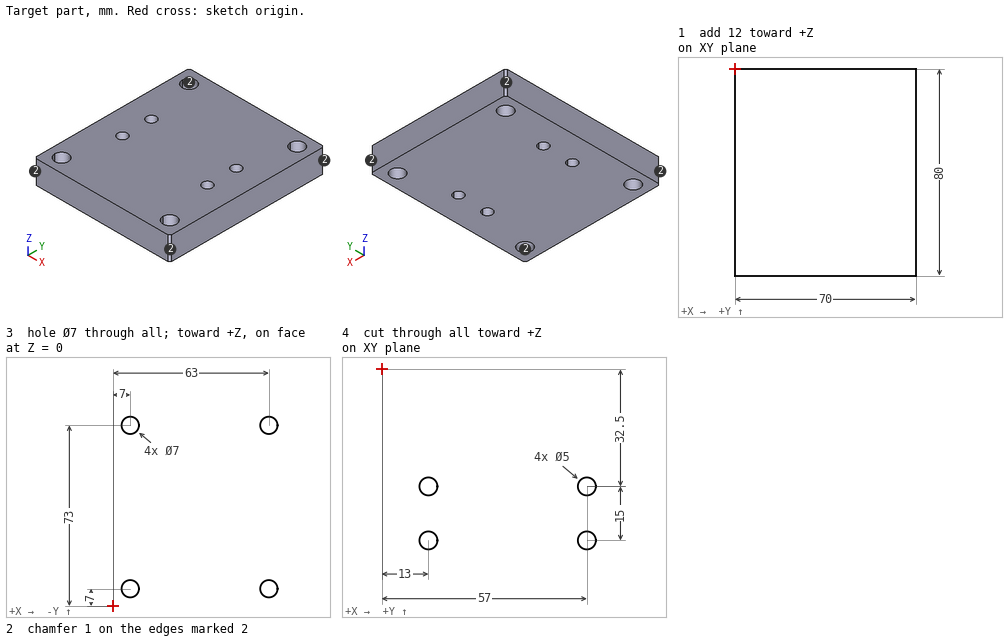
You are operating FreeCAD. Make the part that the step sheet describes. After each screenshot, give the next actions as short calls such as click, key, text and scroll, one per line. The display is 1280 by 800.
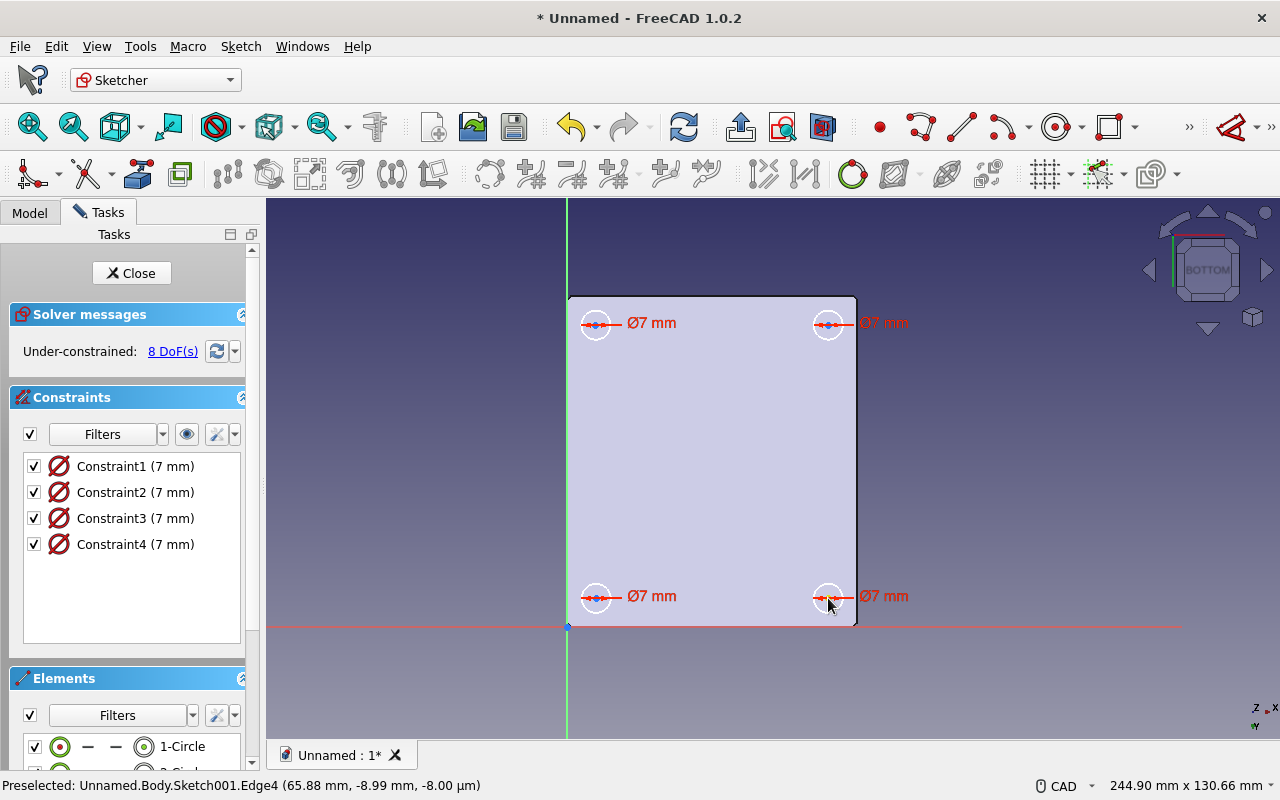
click(596, 325)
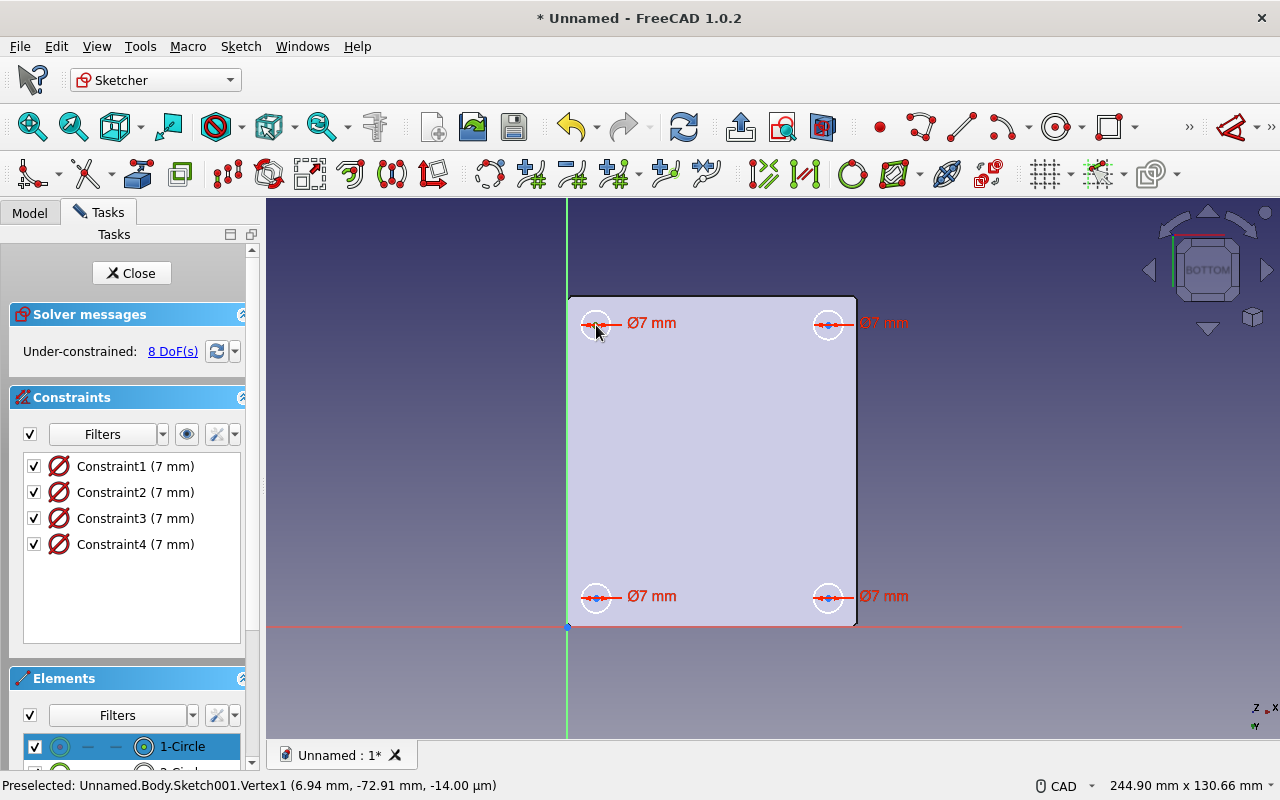
click(596, 598)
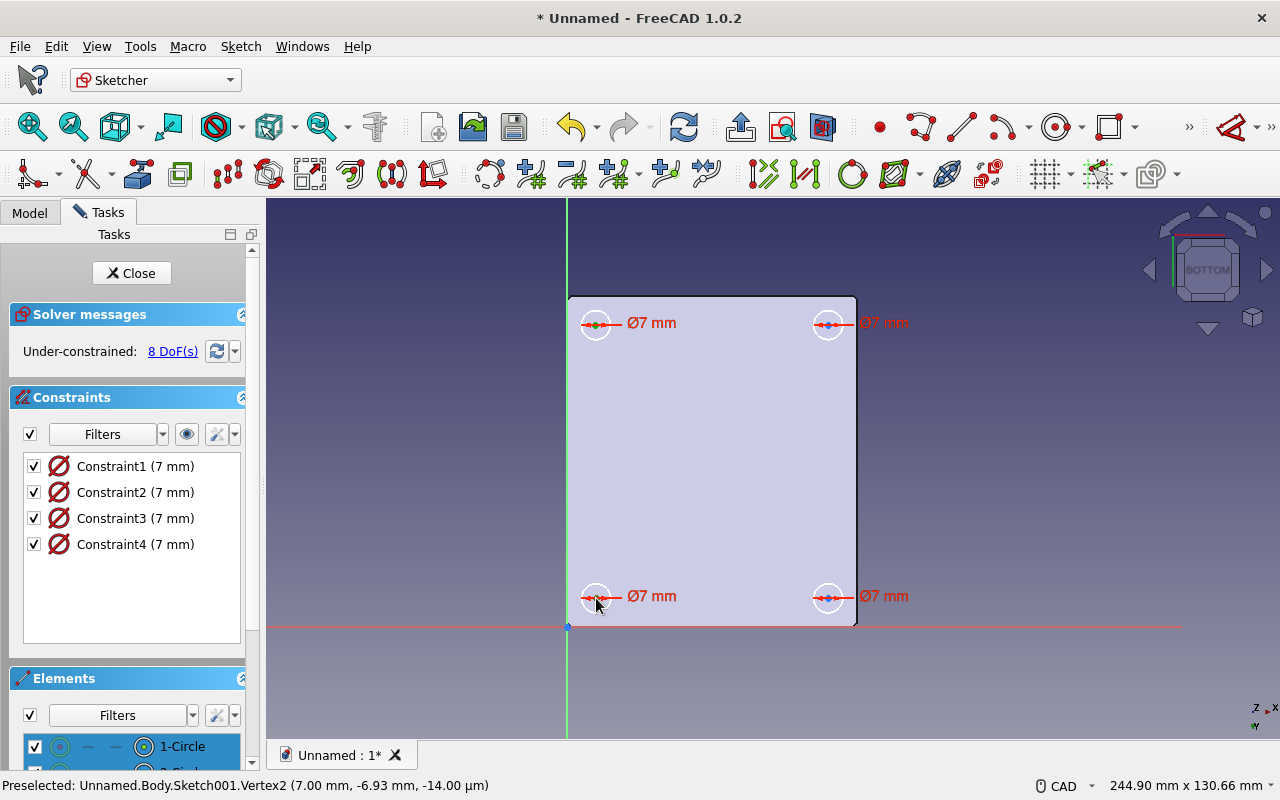
key(v)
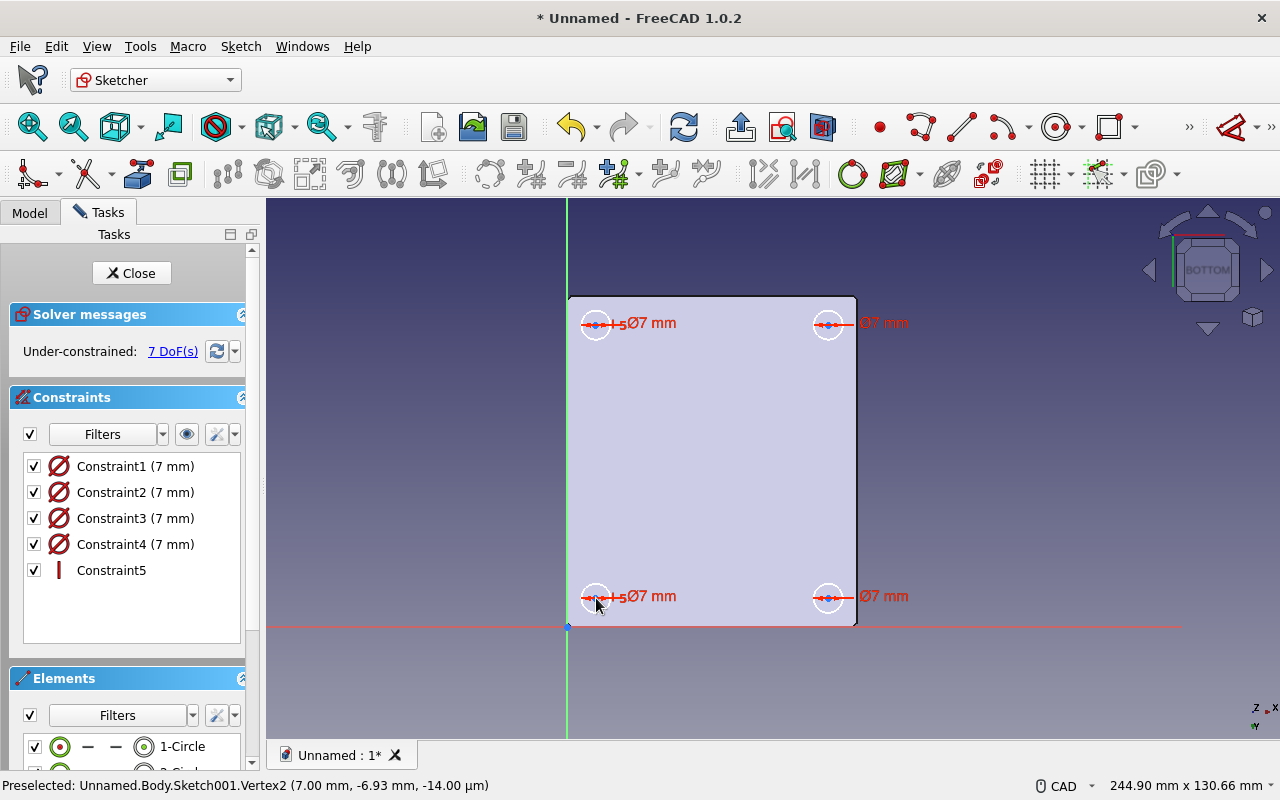
click(596, 325)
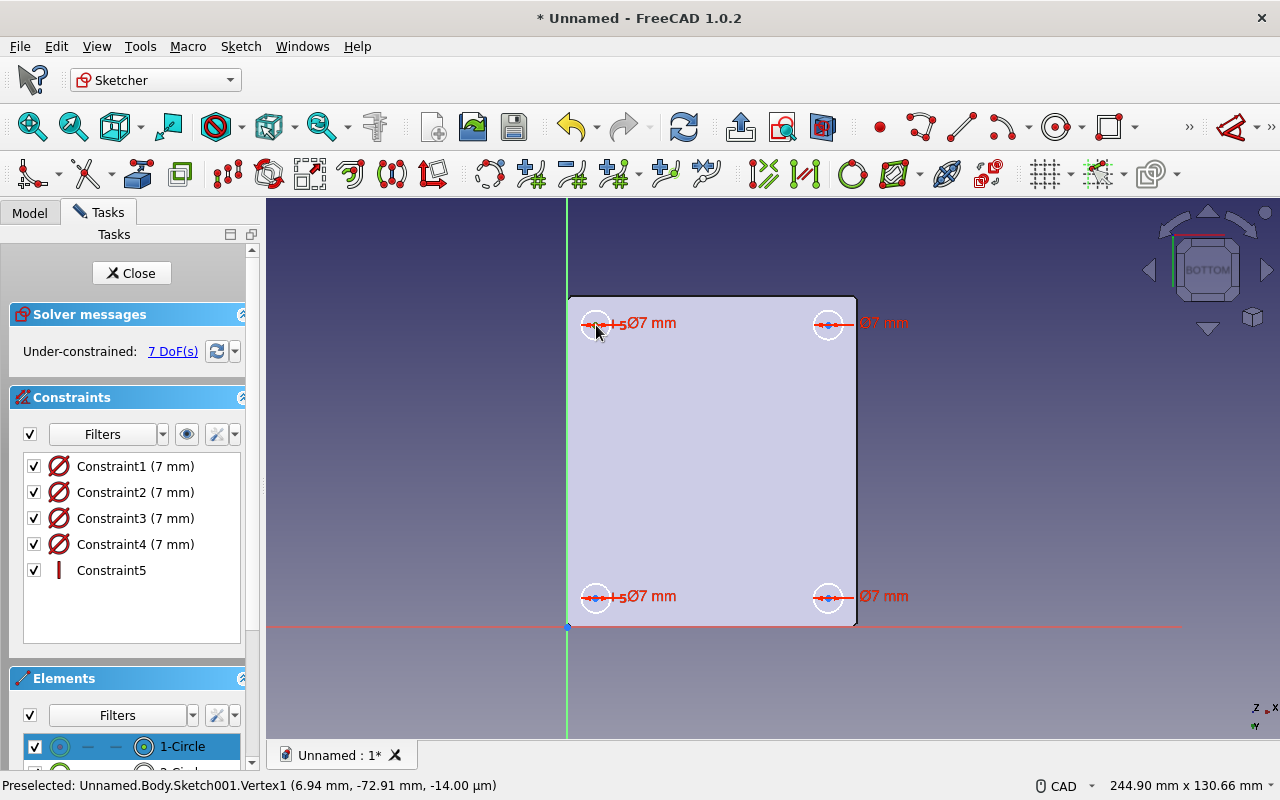
click(828, 325)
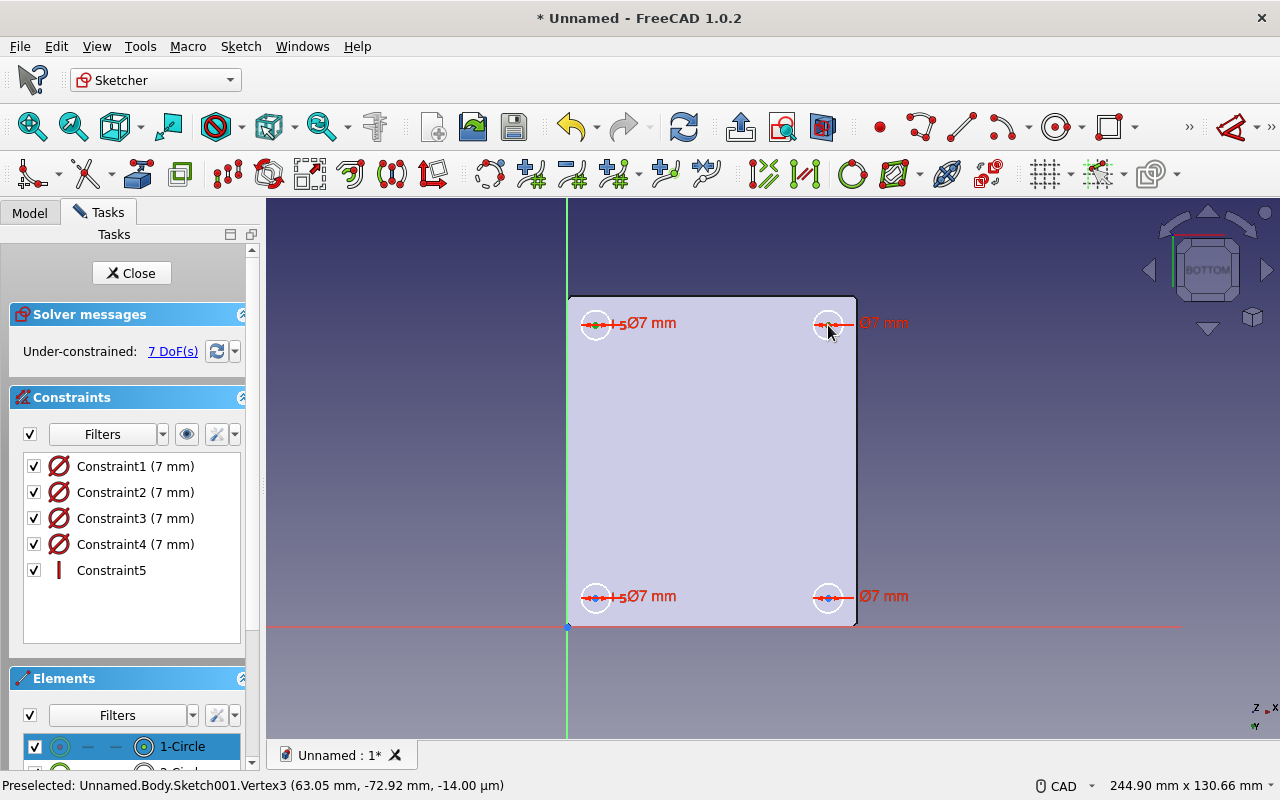
key(h)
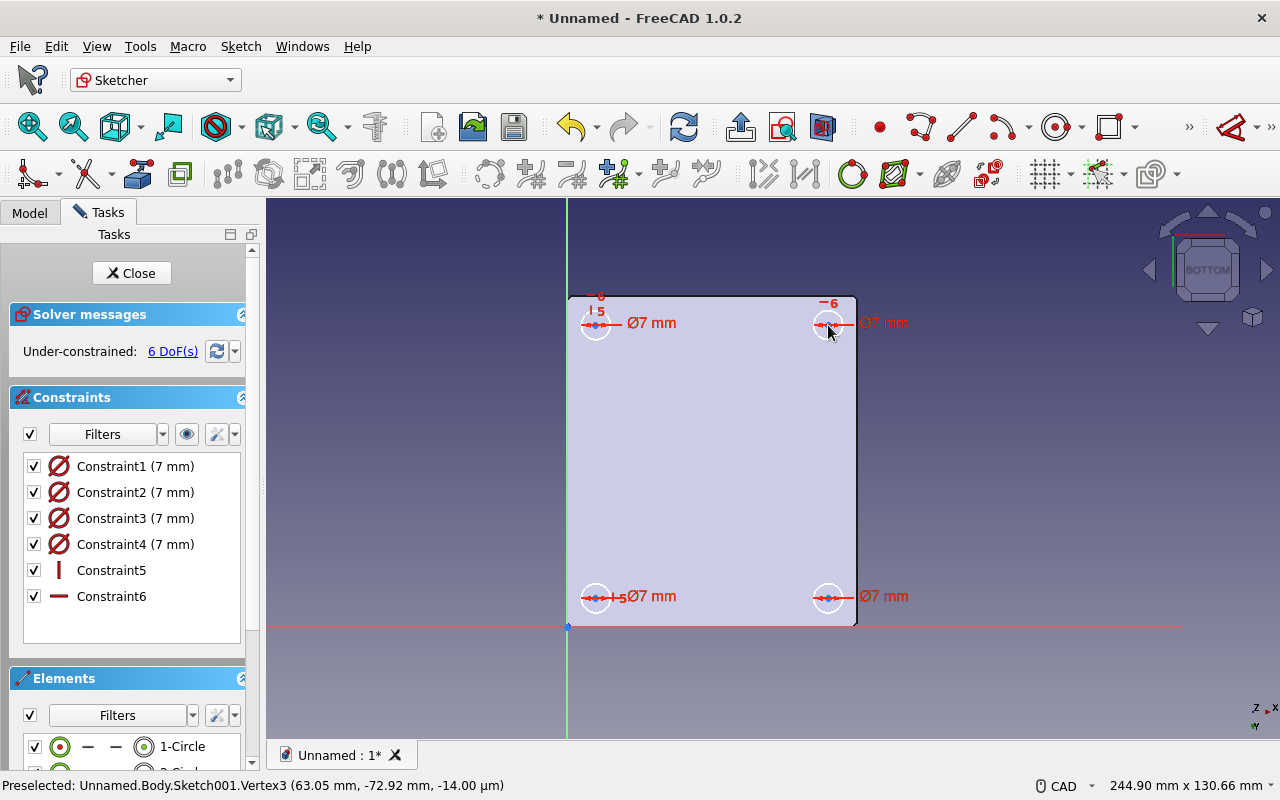
click(828, 325)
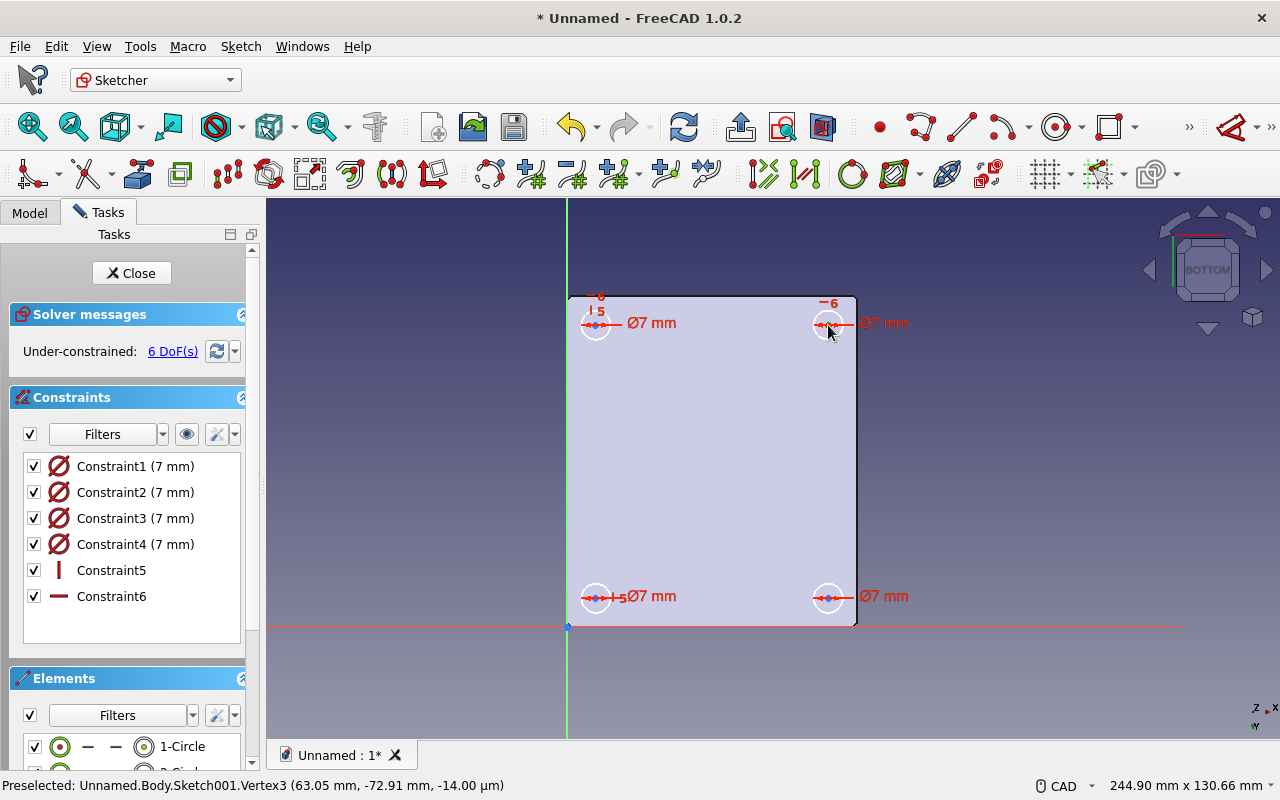
click(828, 598)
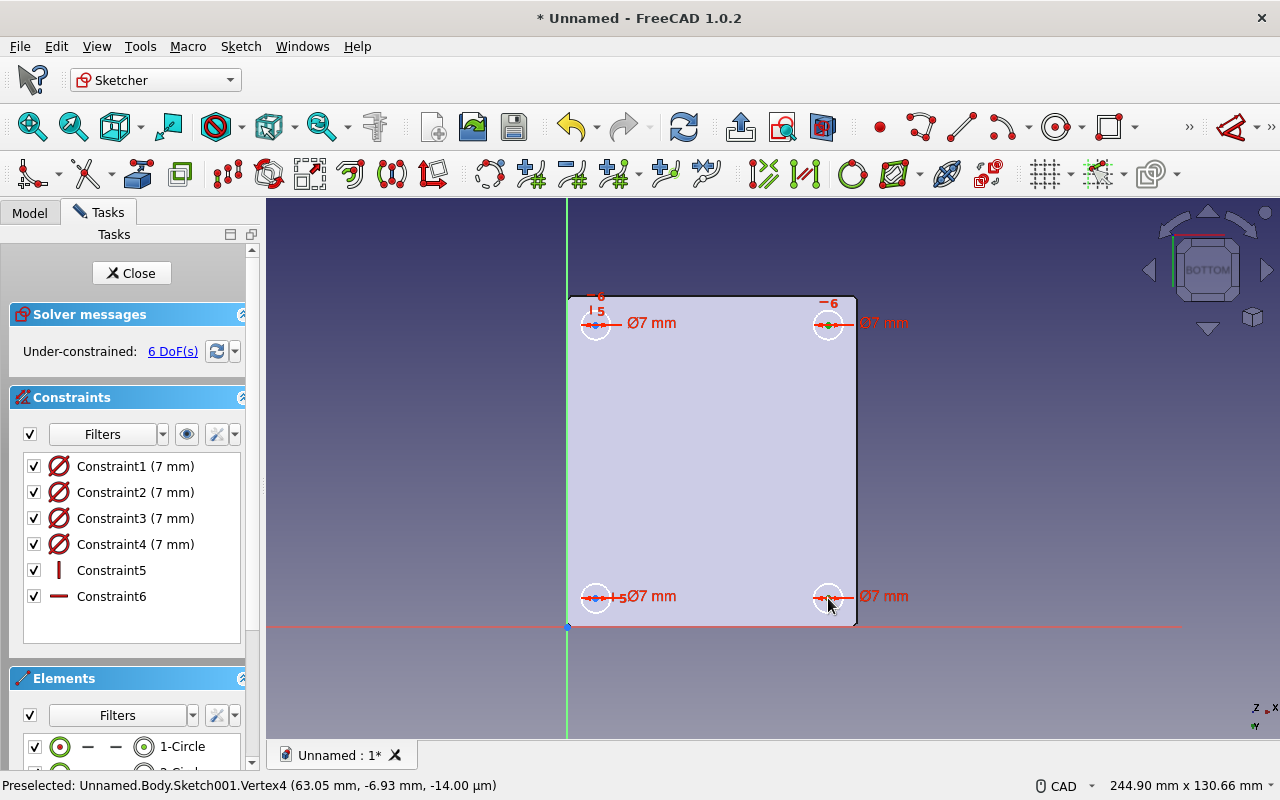
key(v)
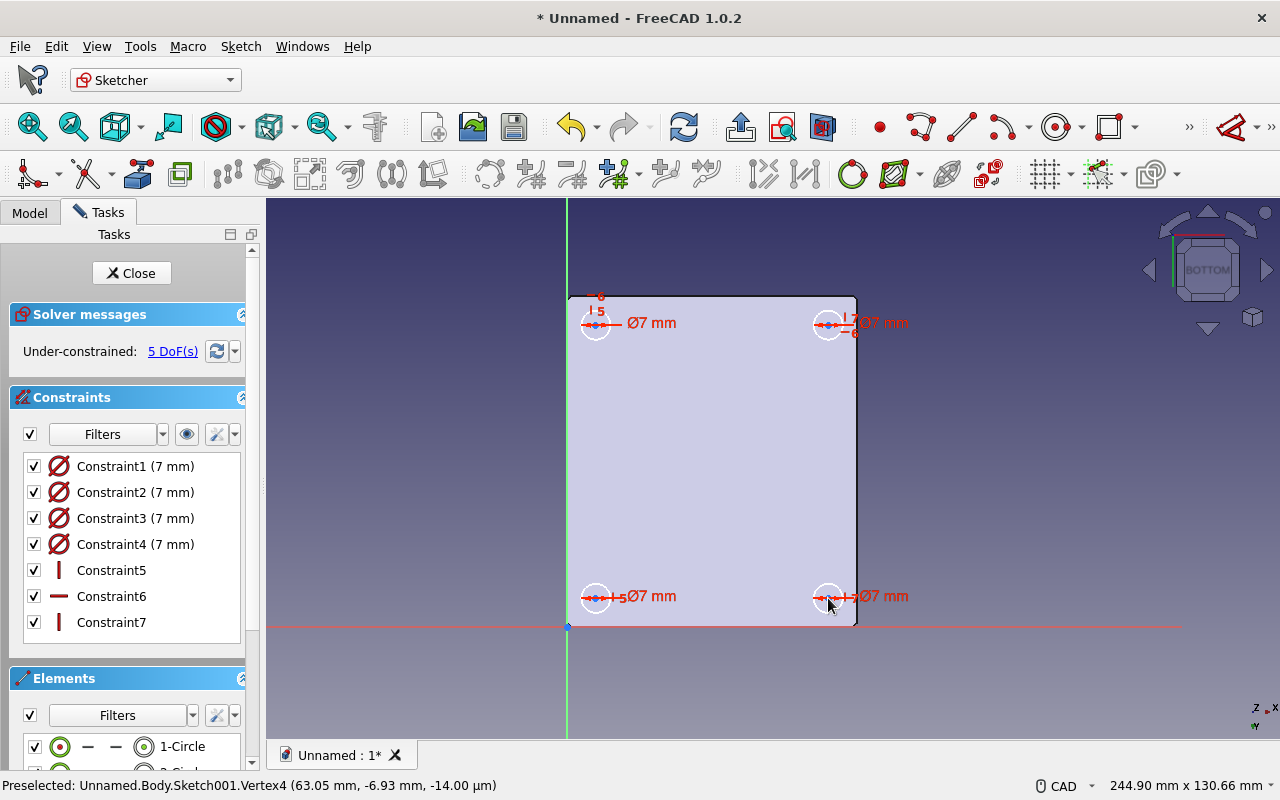
click(596, 598)